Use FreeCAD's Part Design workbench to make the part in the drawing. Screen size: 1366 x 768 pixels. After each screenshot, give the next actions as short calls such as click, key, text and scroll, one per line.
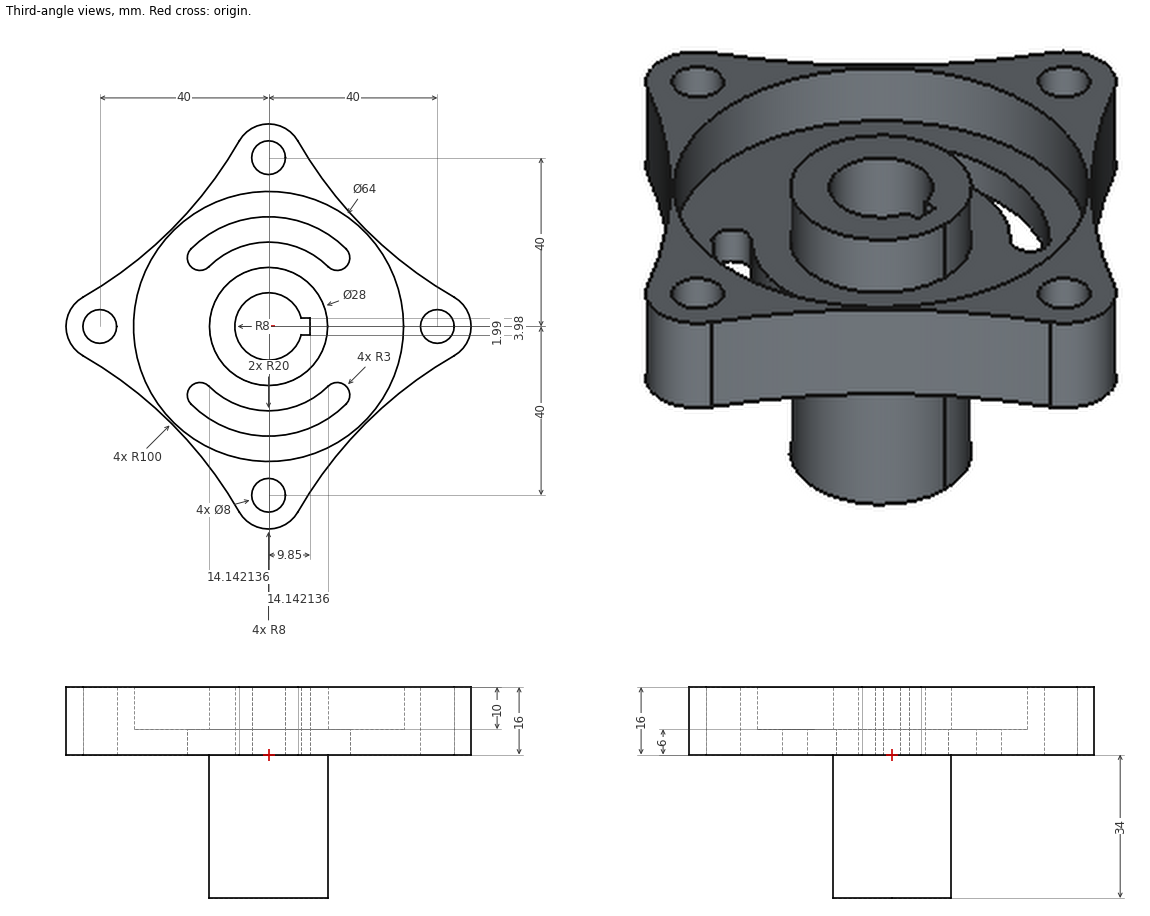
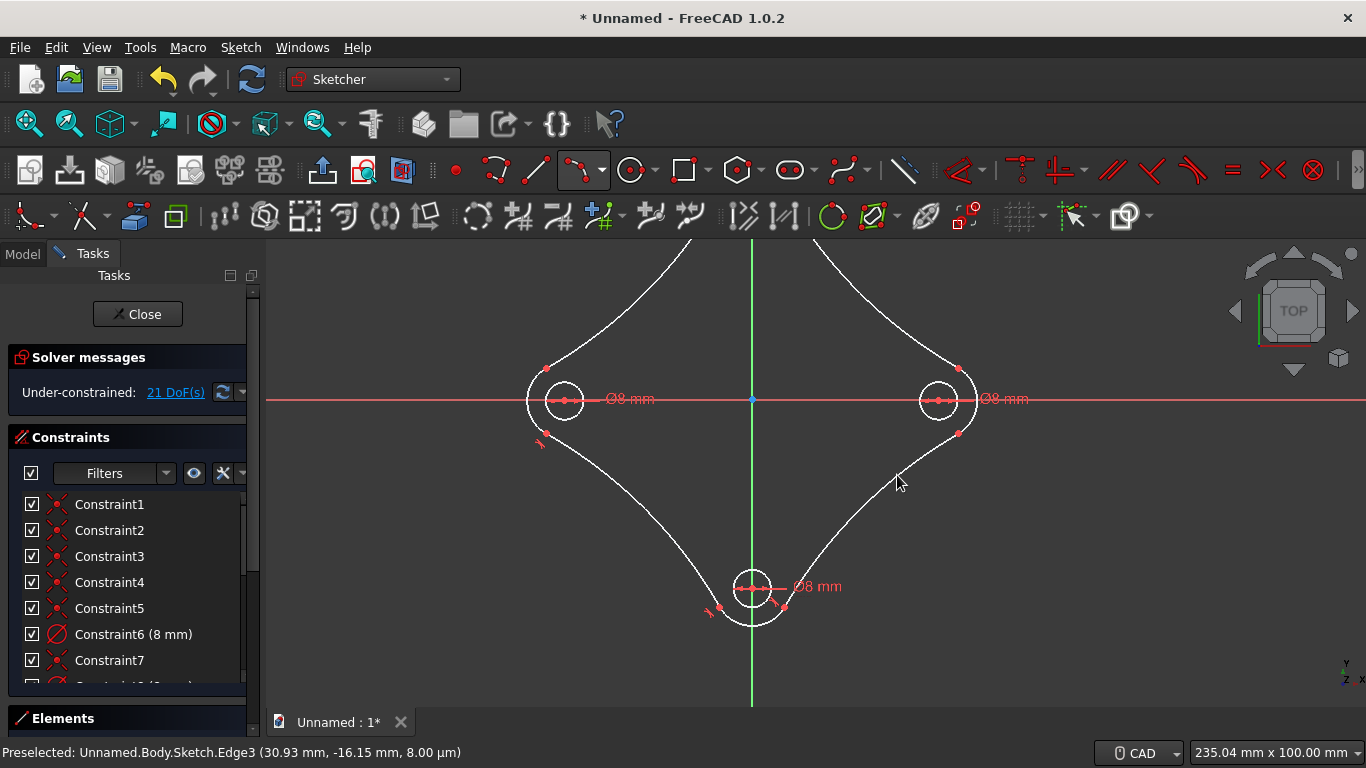
click(897, 476)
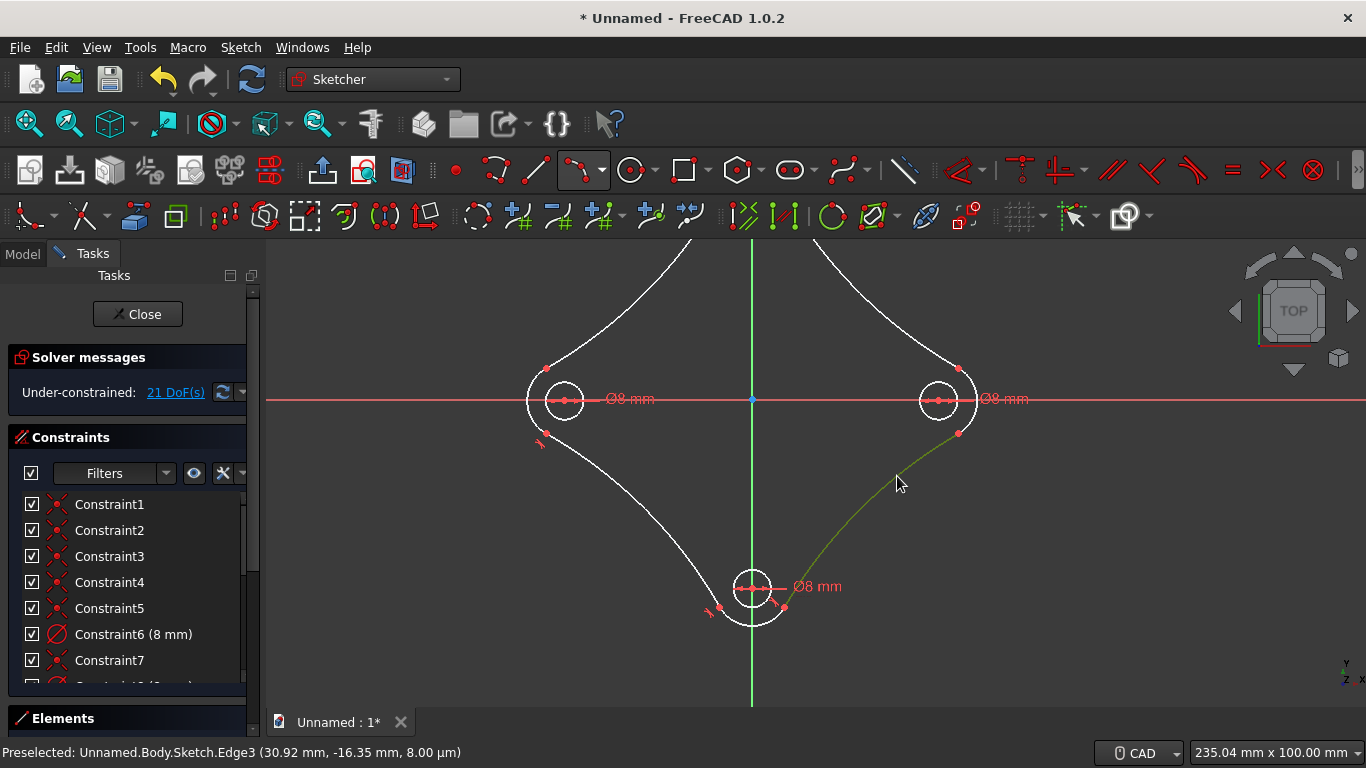
click(974, 416)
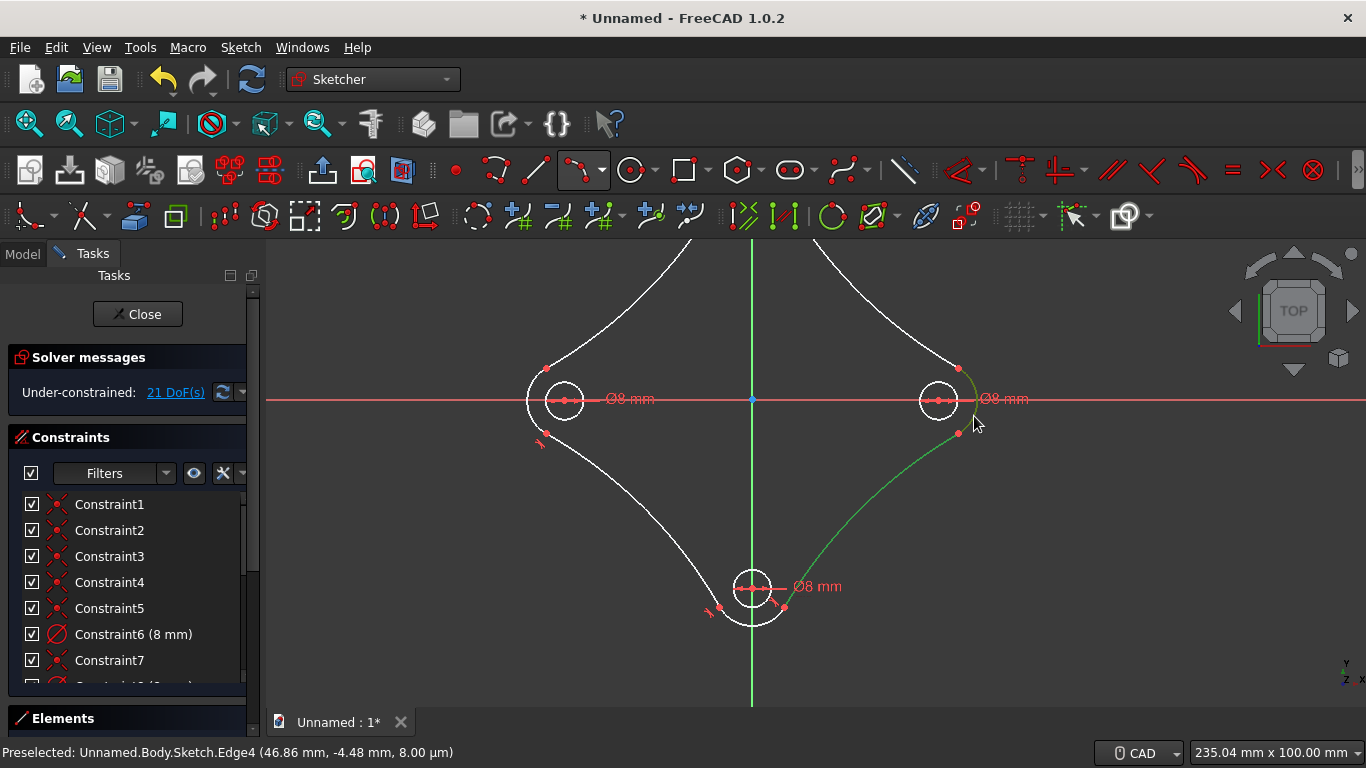
key(t)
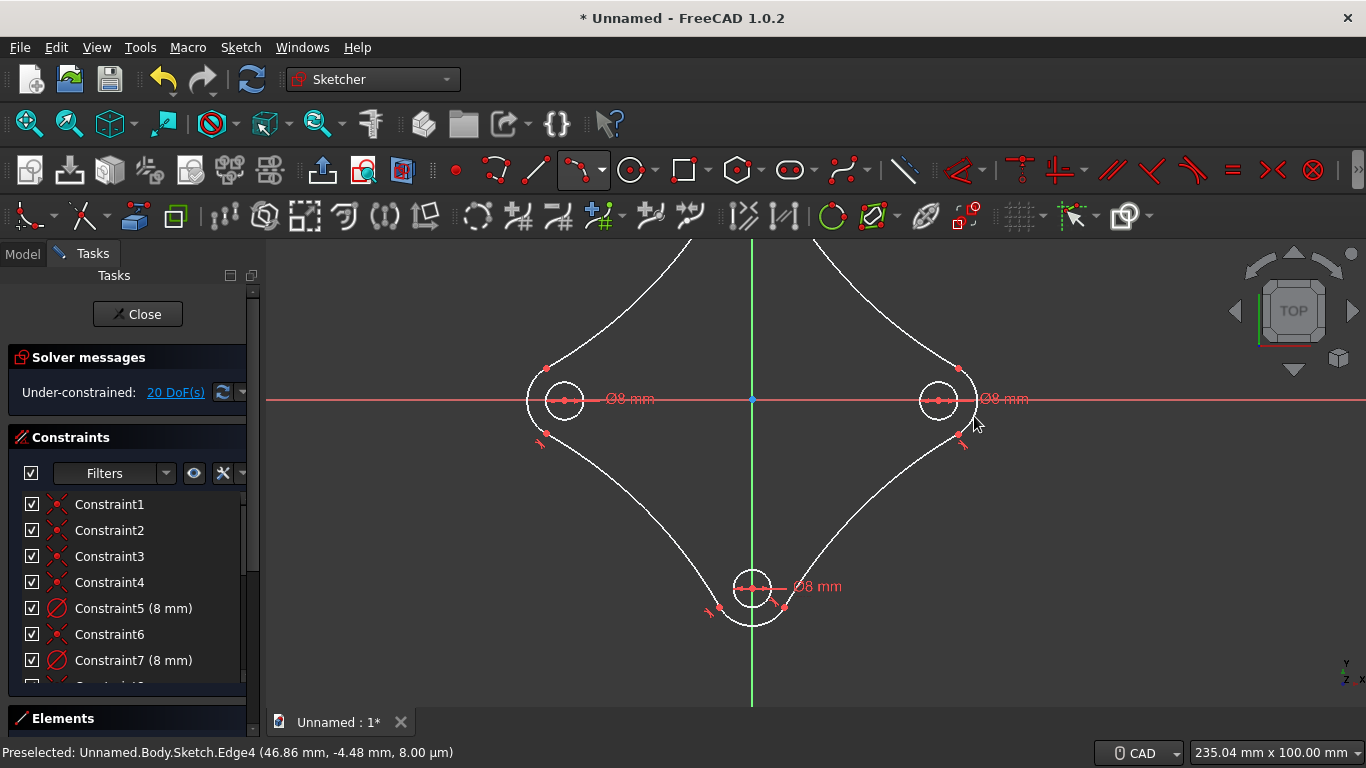
click(974, 417)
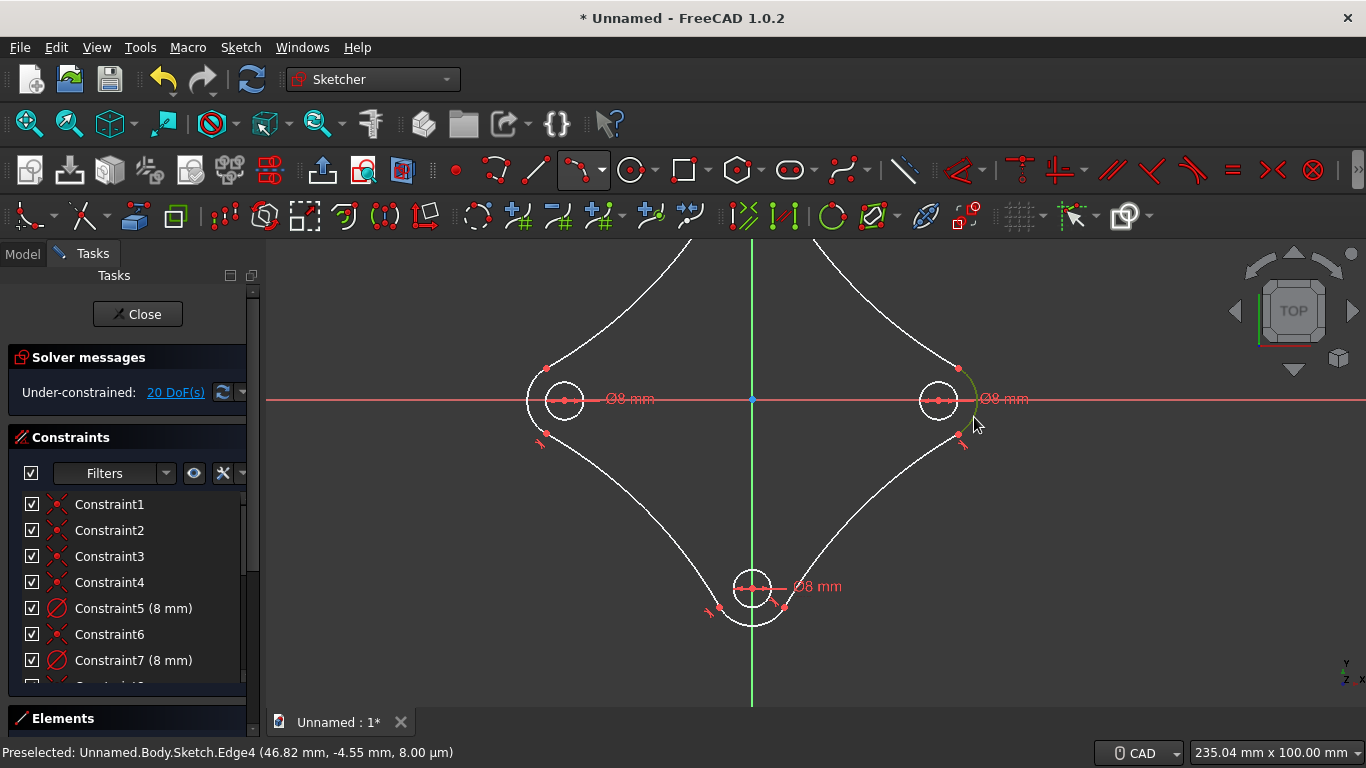
click(897, 326)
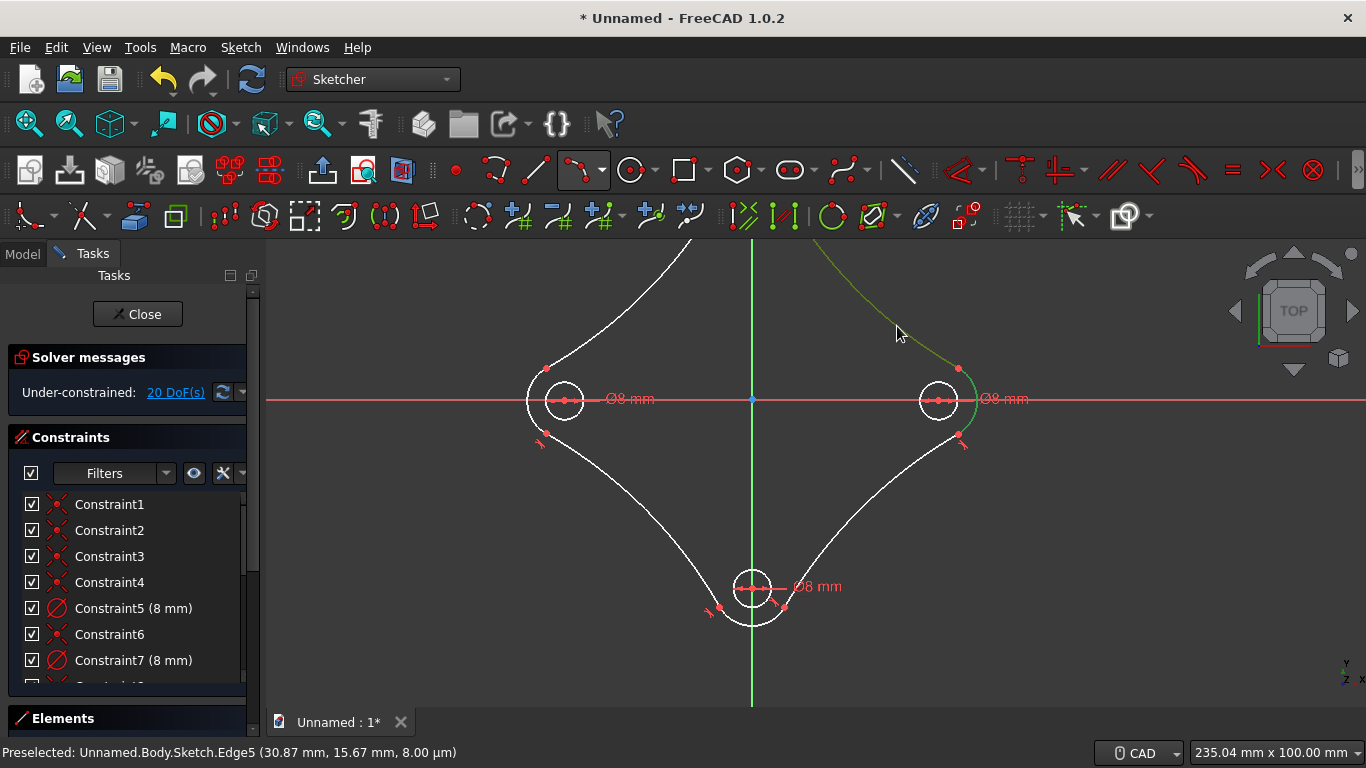
click(1194, 170)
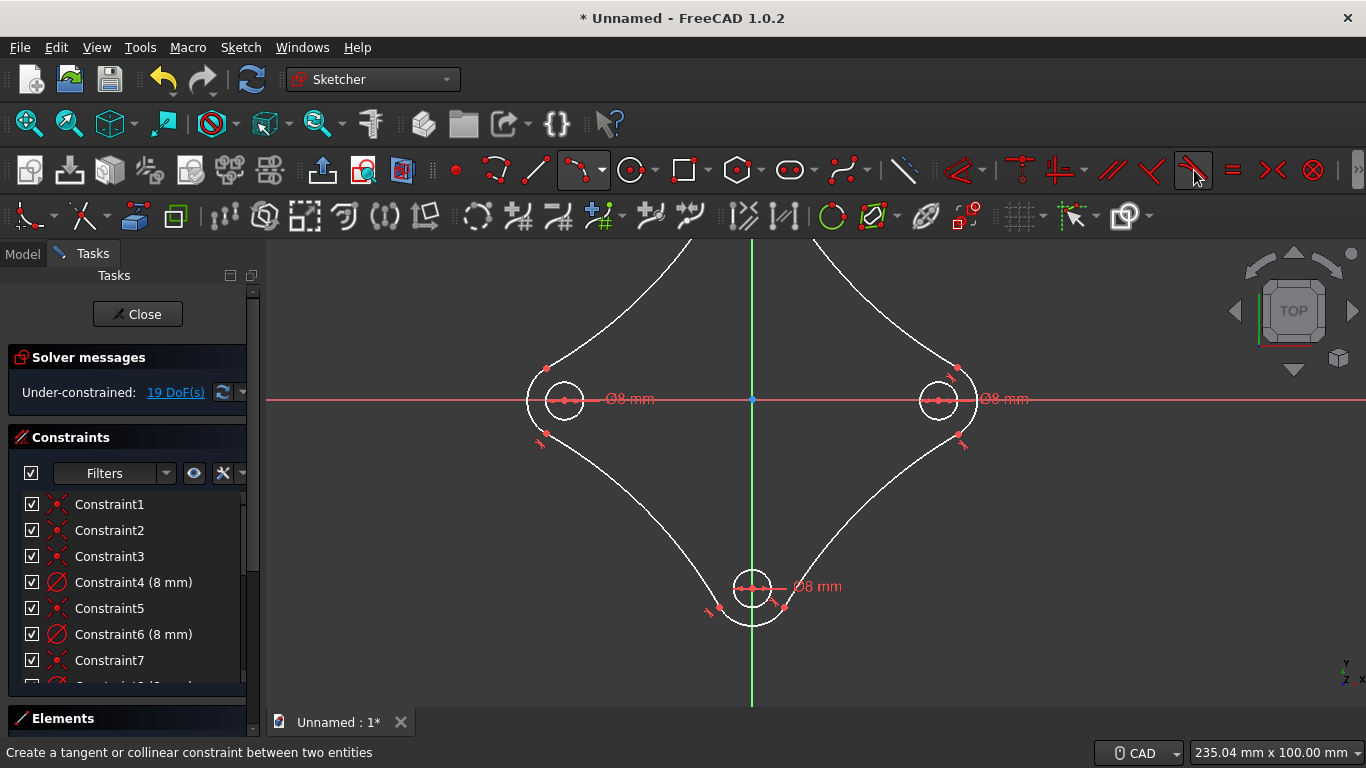
click(896, 326)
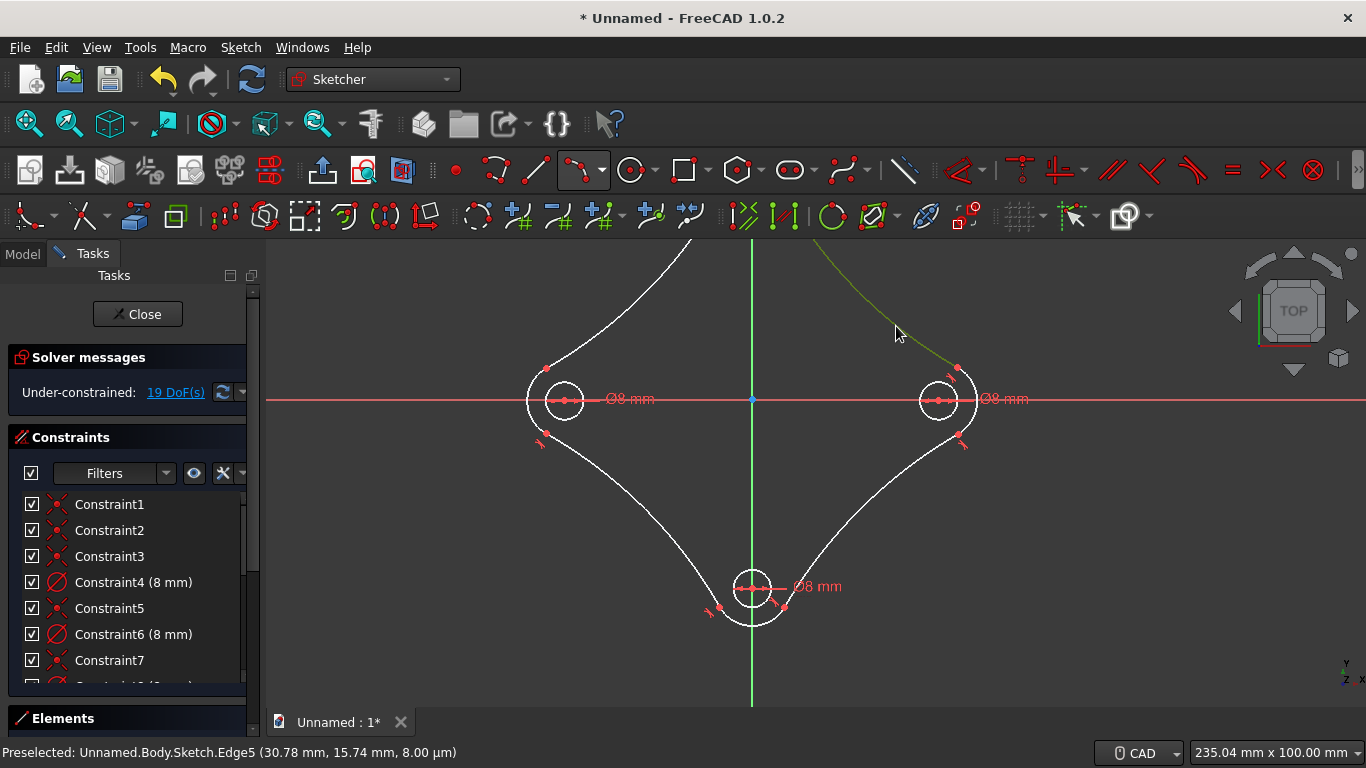
scroll(737, 622, down, 2)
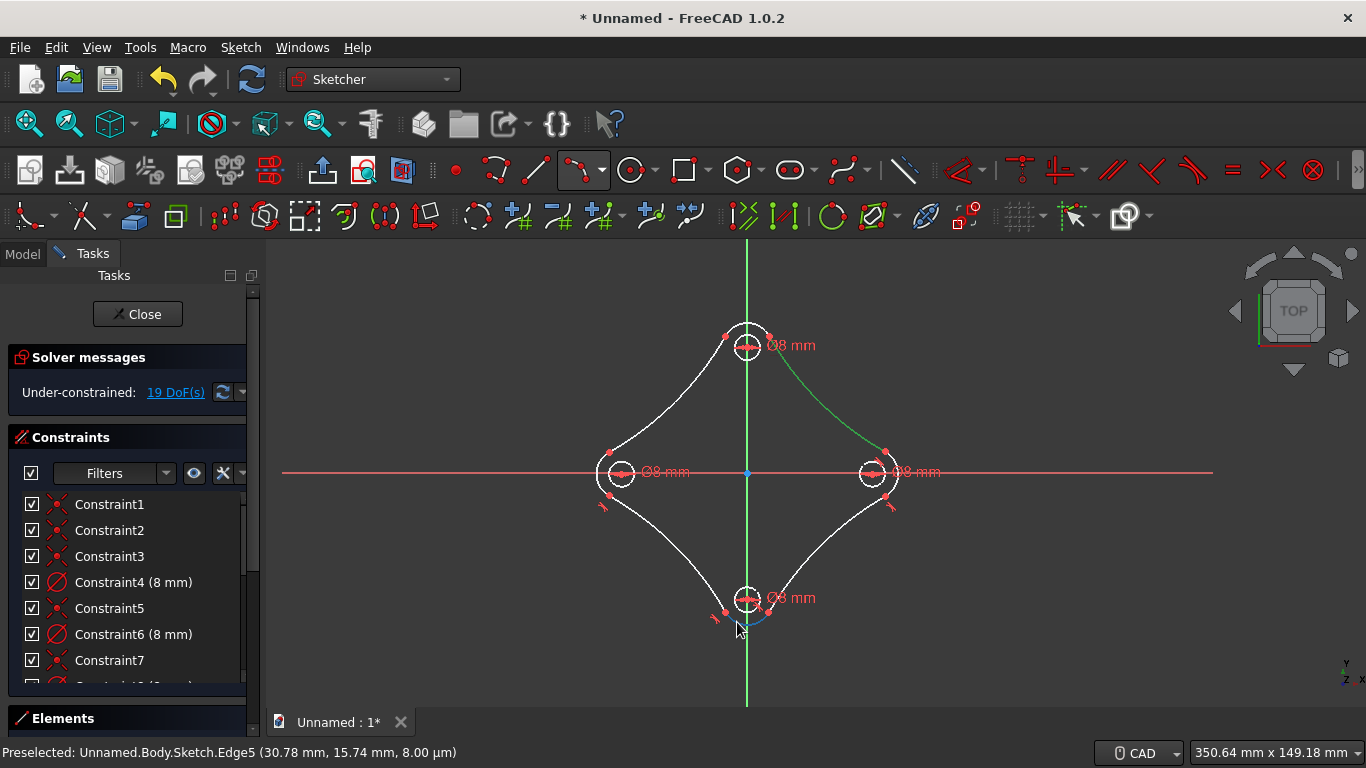
scroll(758, 325, up, 2)